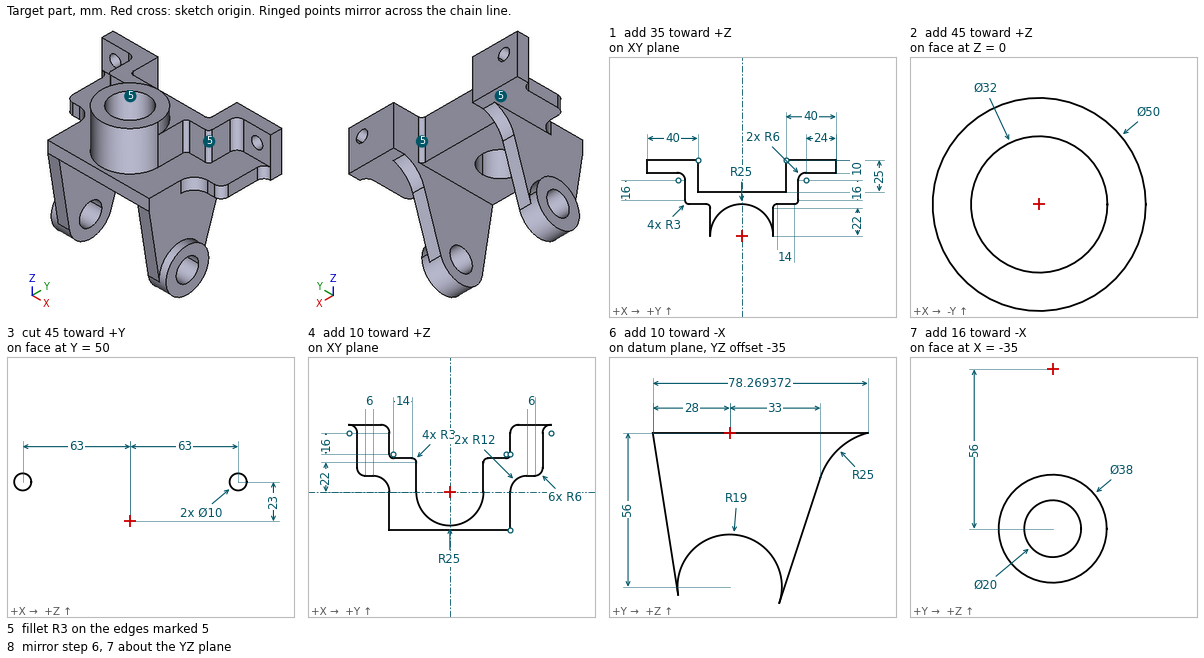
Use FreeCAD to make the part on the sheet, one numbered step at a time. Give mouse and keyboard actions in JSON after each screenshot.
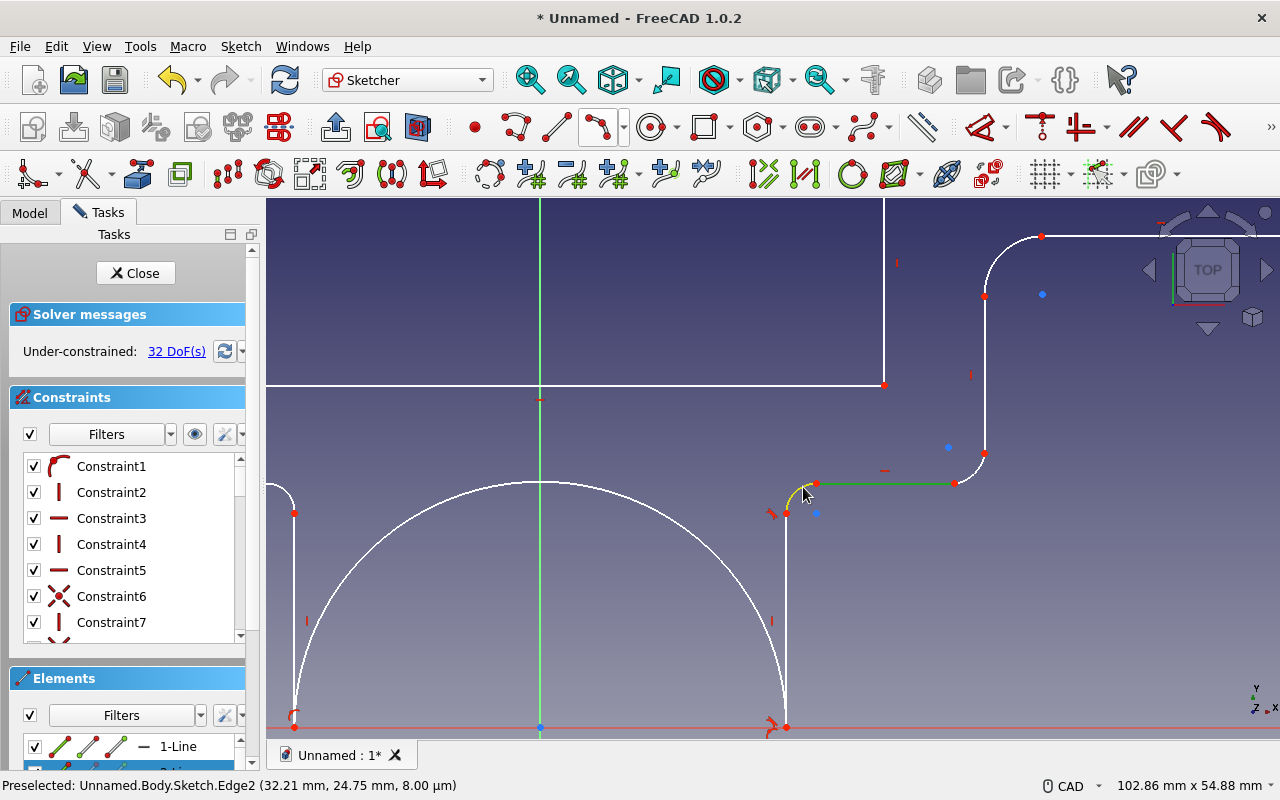
{"action": "left_click", "coordinate": [803, 487]}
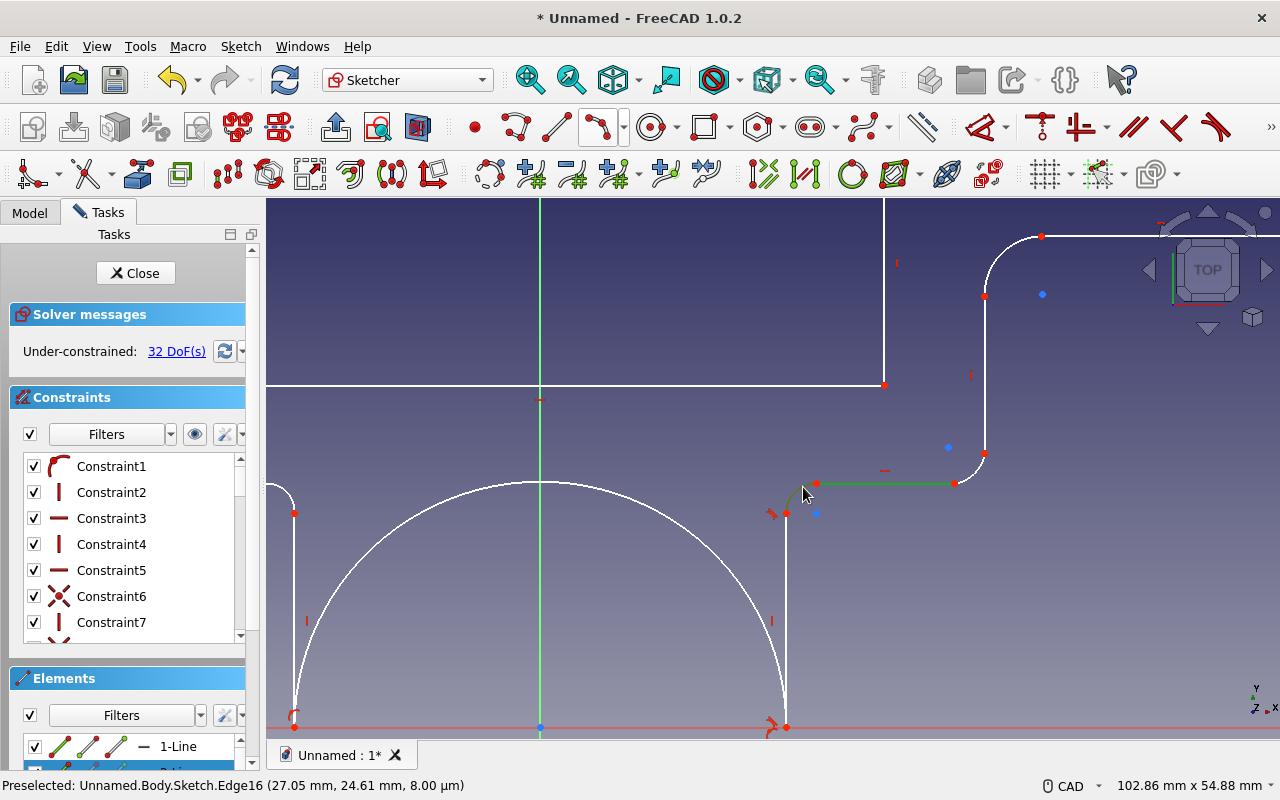
{"action": "left_click", "coordinate": [1216, 128]}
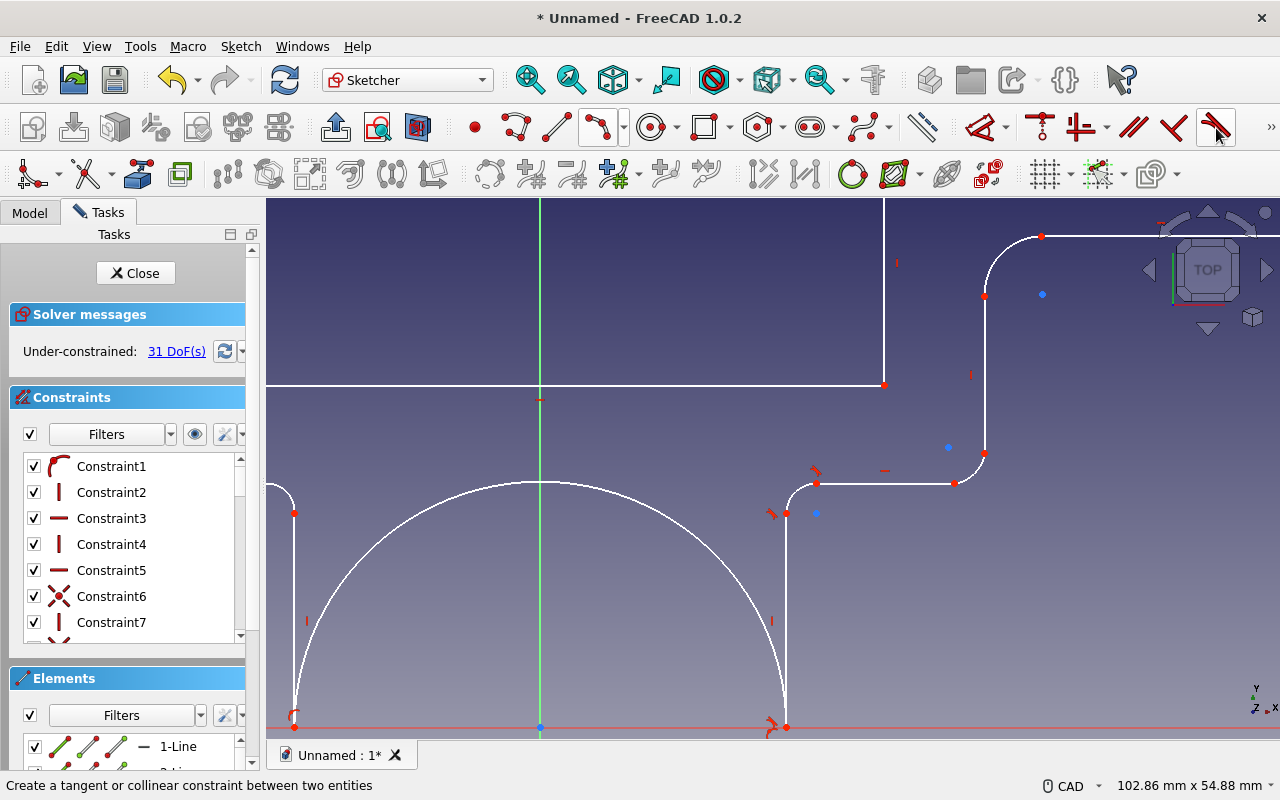
{"action": "left_click", "coordinate": [858, 484]}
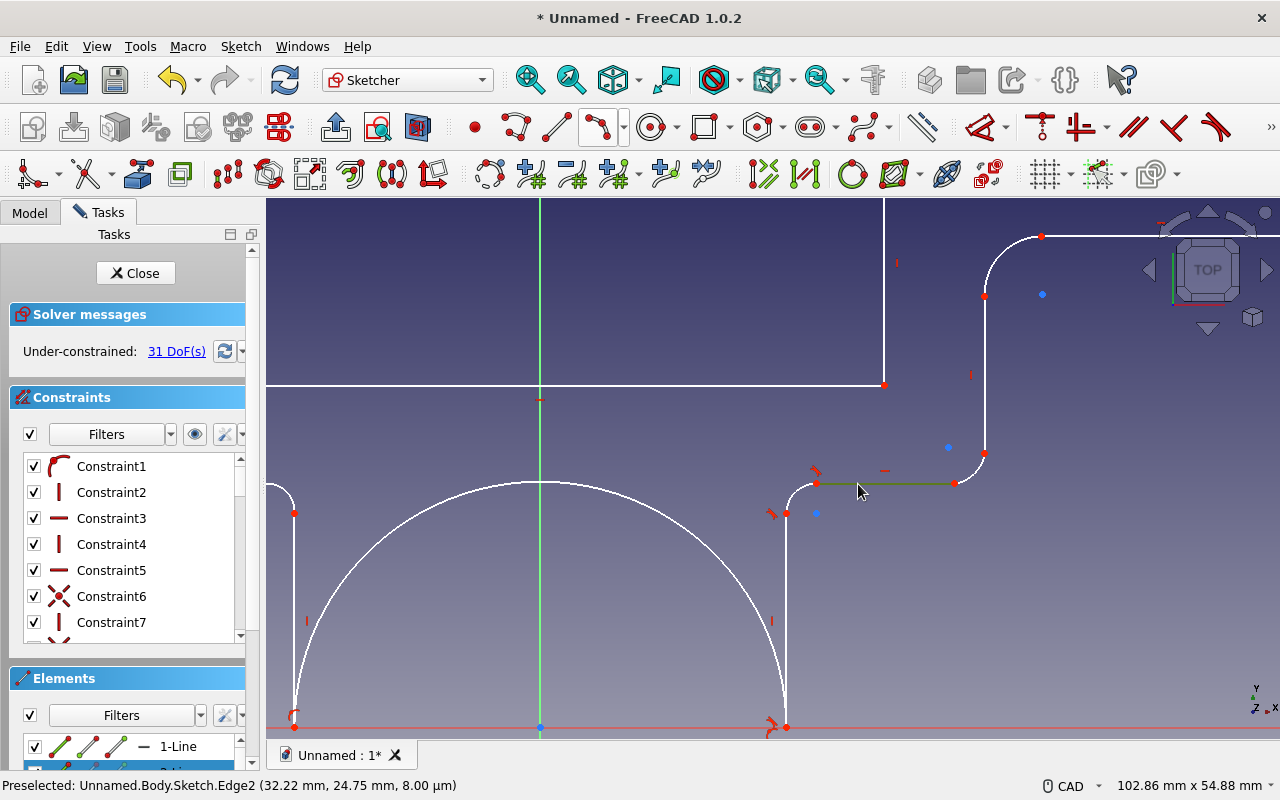
{"action": "left_click", "coordinate": [967, 479]}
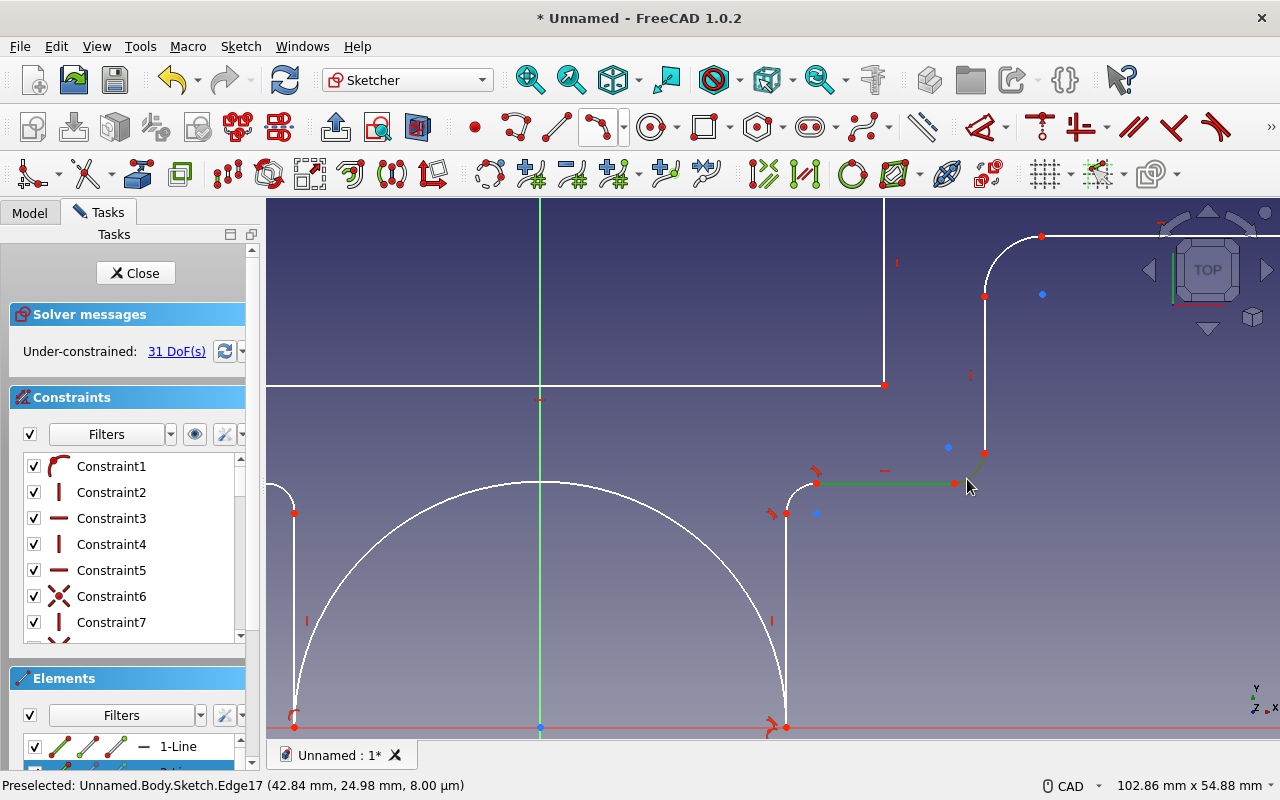
{"action": "left_click", "coordinate": [1216, 128]}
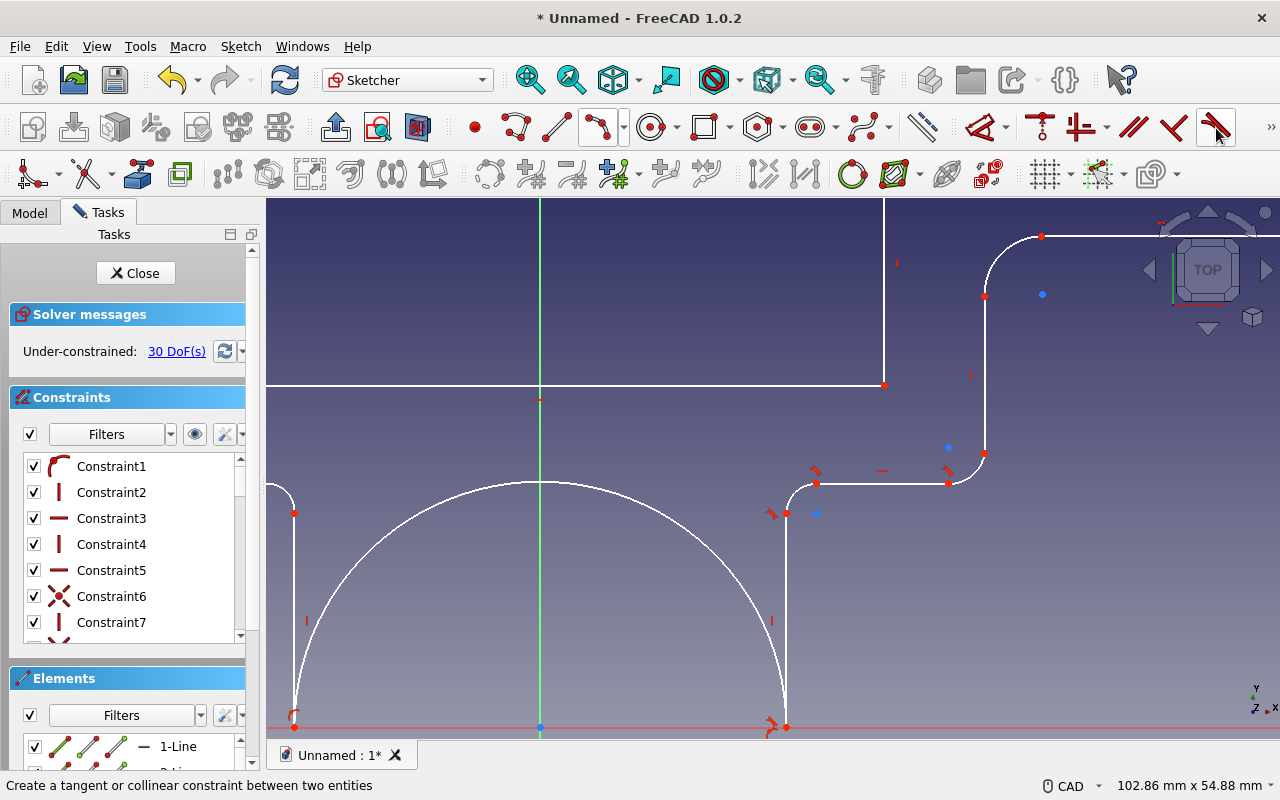
{"action": "left_click", "coordinate": [985, 407]}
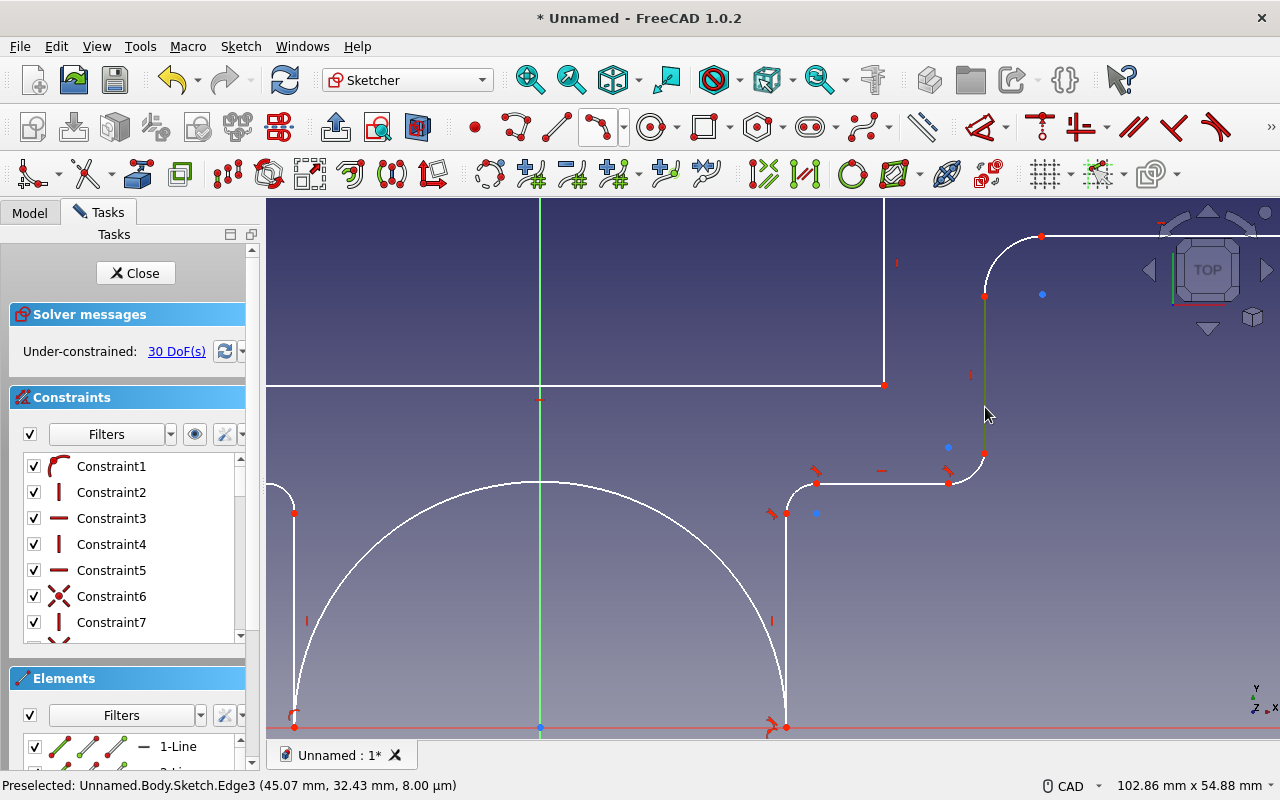
{"action": "left_click", "coordinate": [964, 481]}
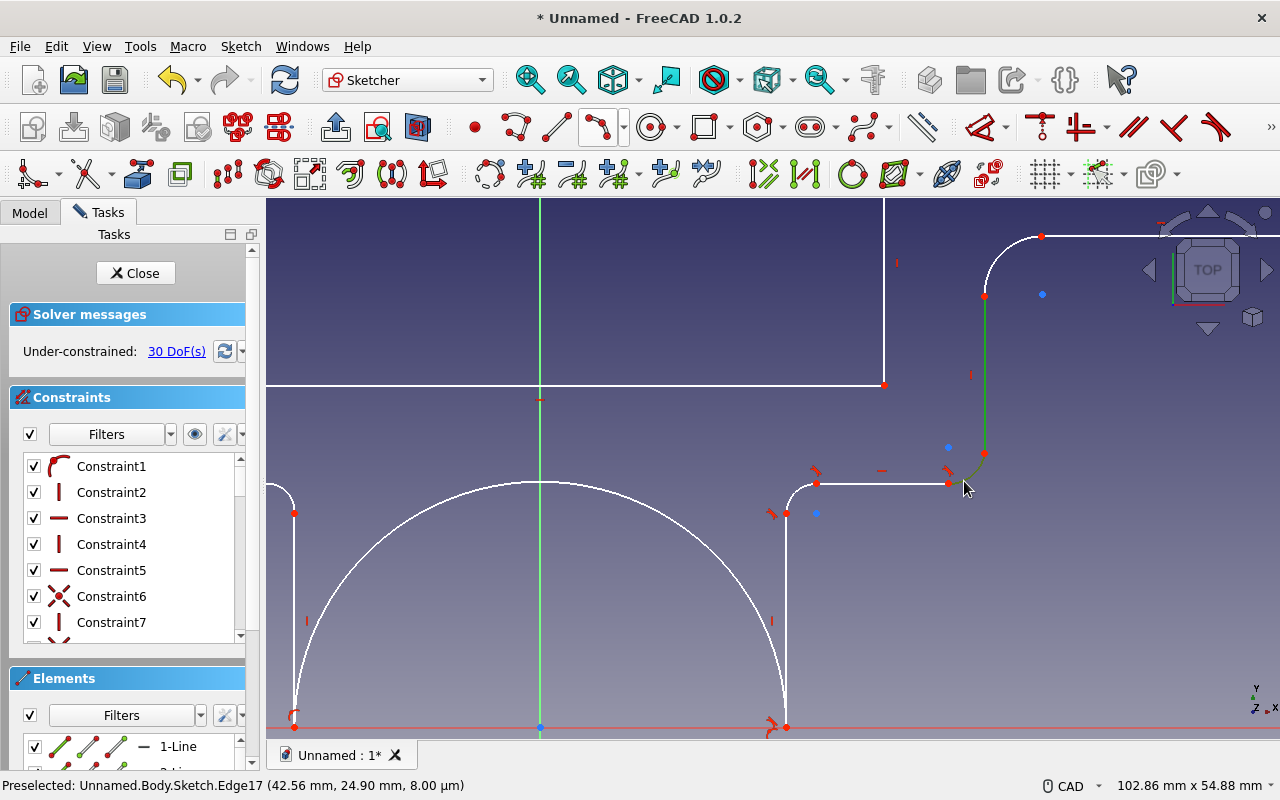
{"action": "left_click", "coordinate": [1216, 128]}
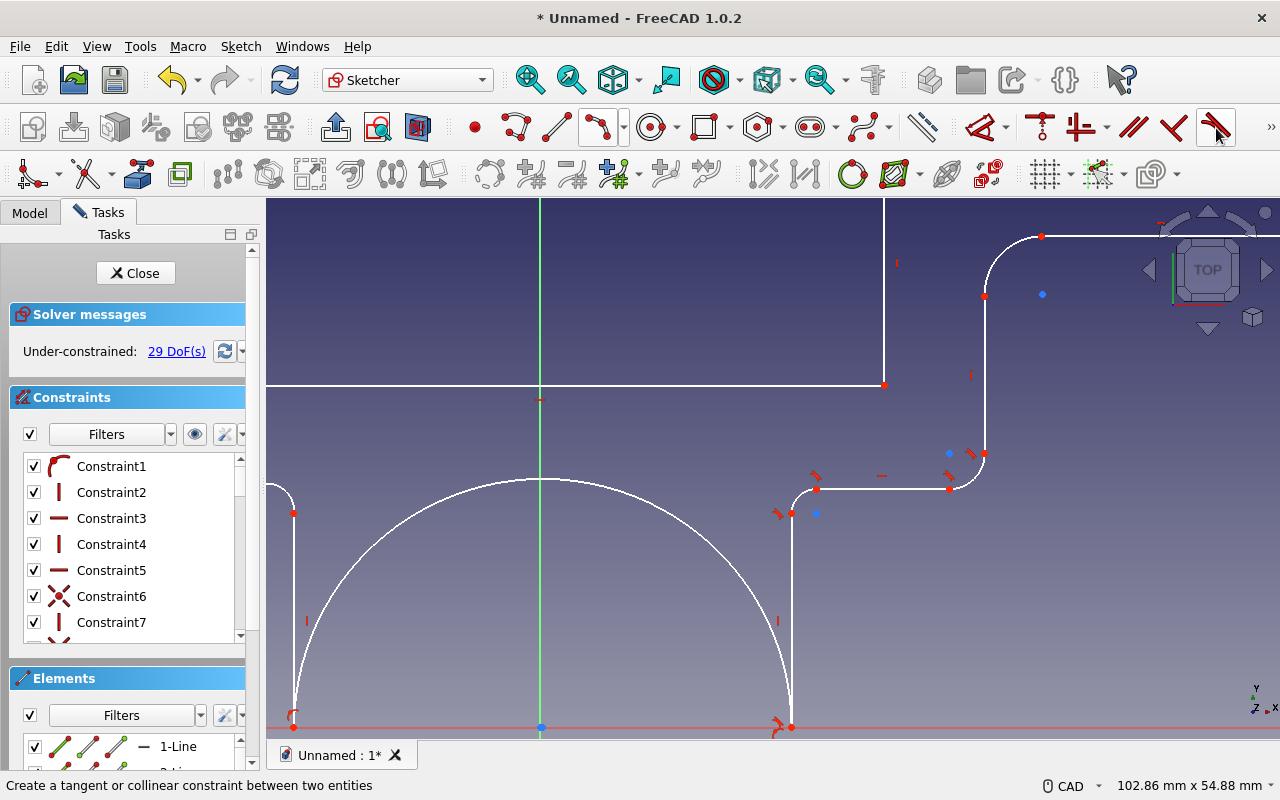
{"action": "left_click", "coordinate": [985, 406]}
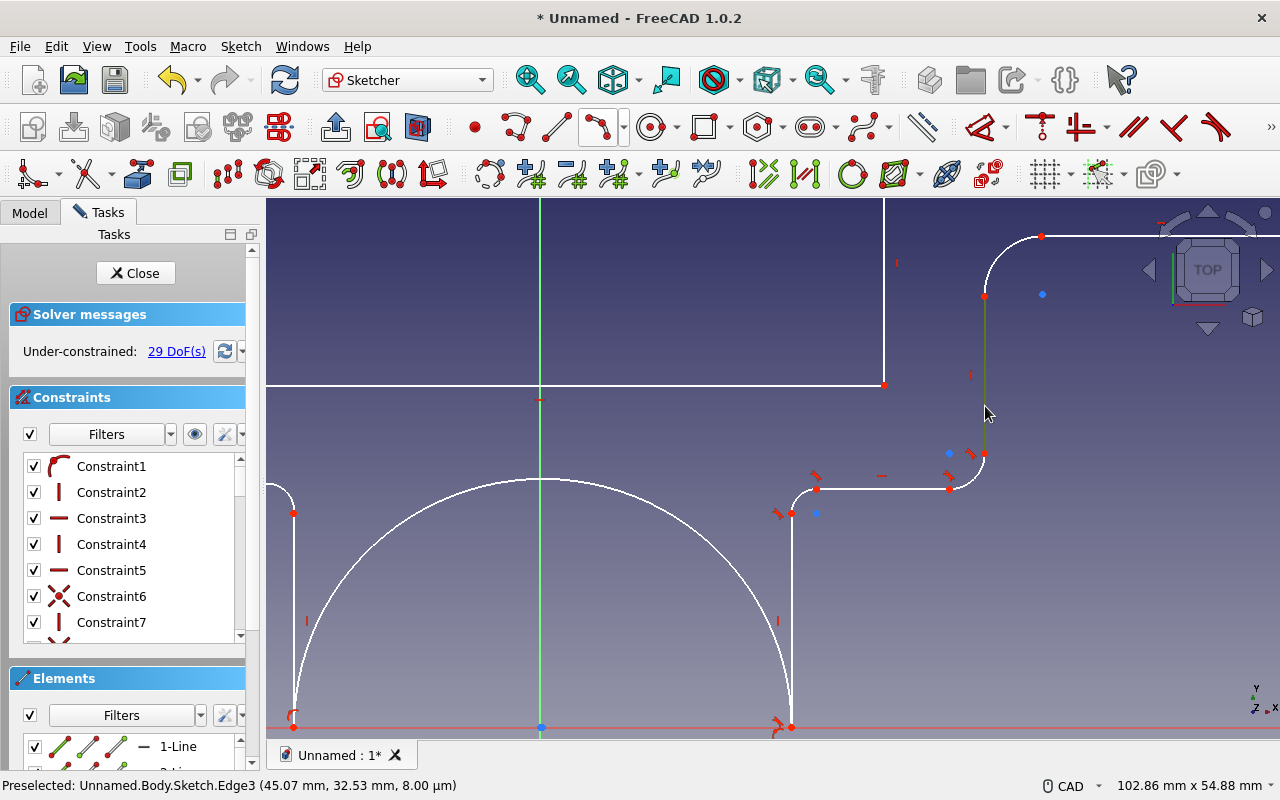
{"action": "left_click", "coordinate": [1015, 243]}